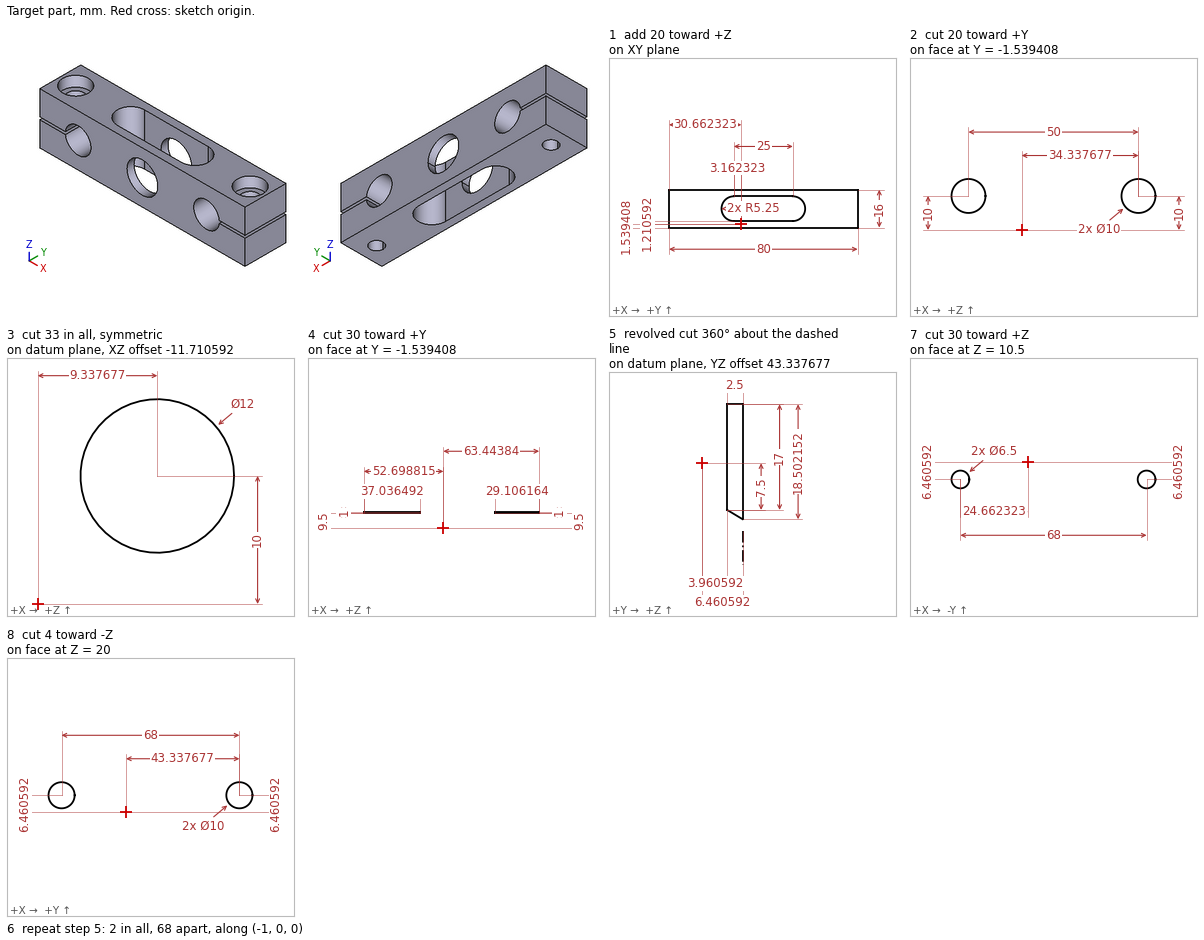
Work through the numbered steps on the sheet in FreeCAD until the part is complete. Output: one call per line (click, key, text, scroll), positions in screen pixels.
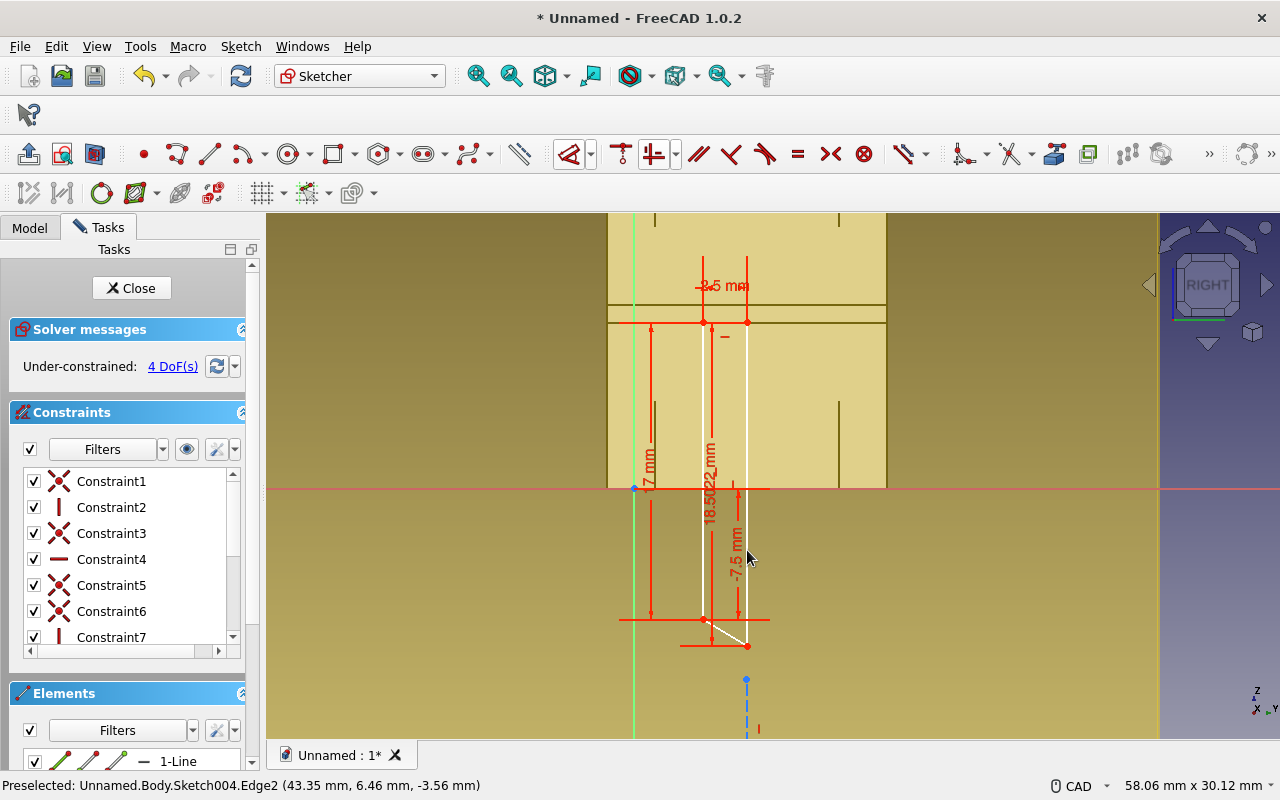
click(703, 620)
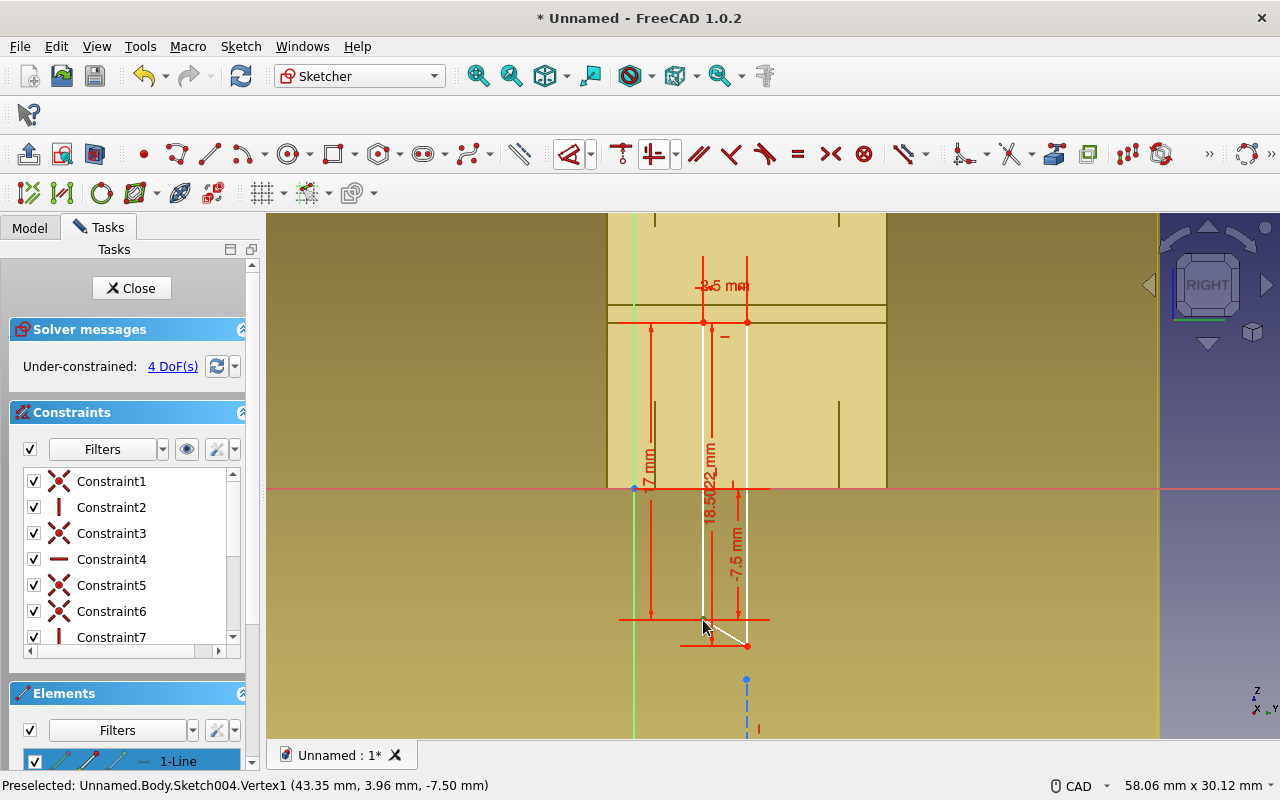
click(590, 154)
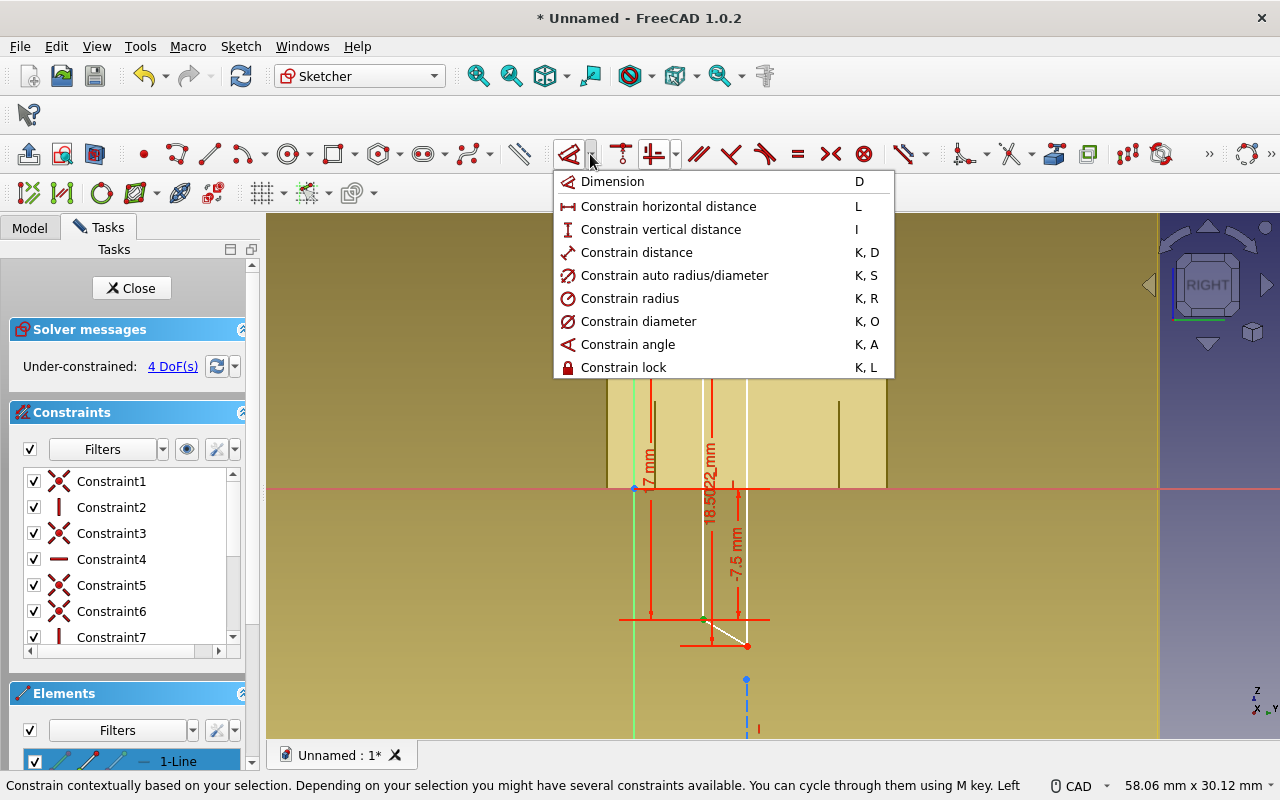
click(724, 206)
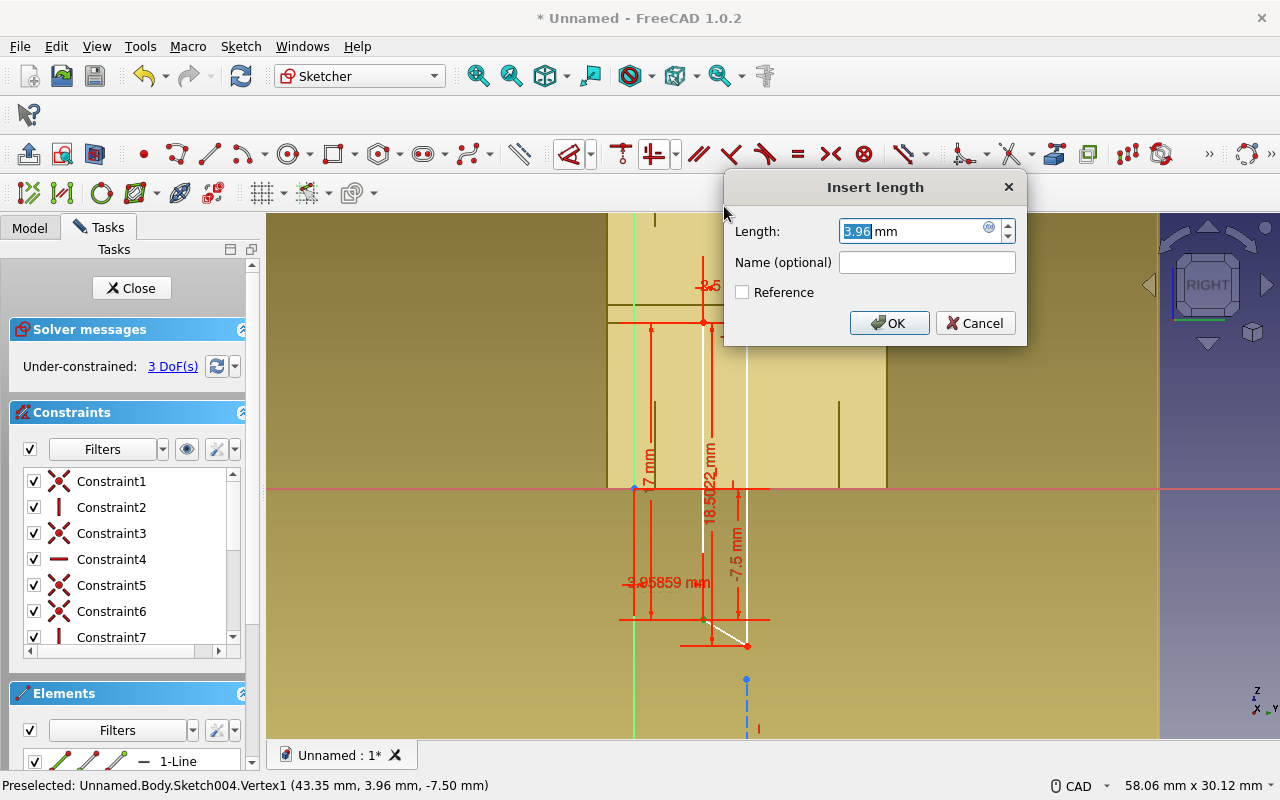
text(3.960592)
key(Return)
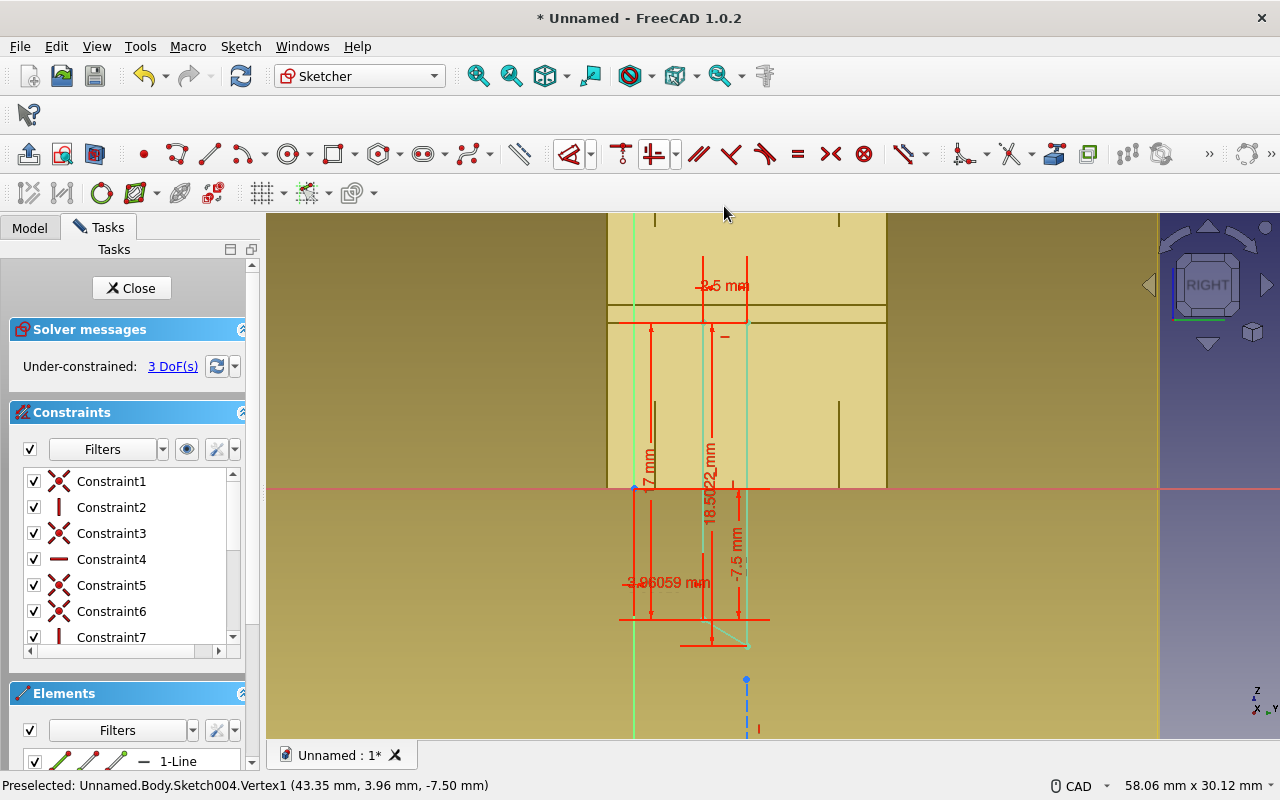
click(747, 680)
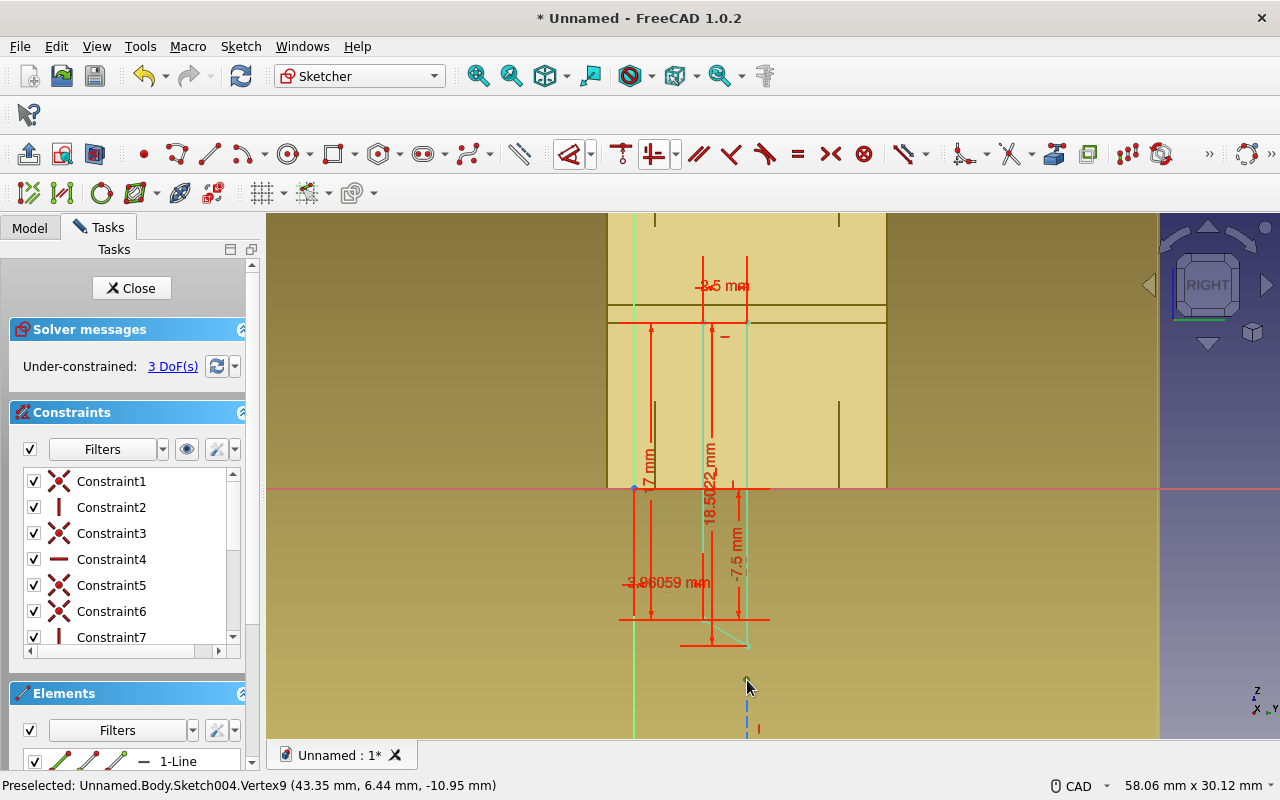
click(590, 154)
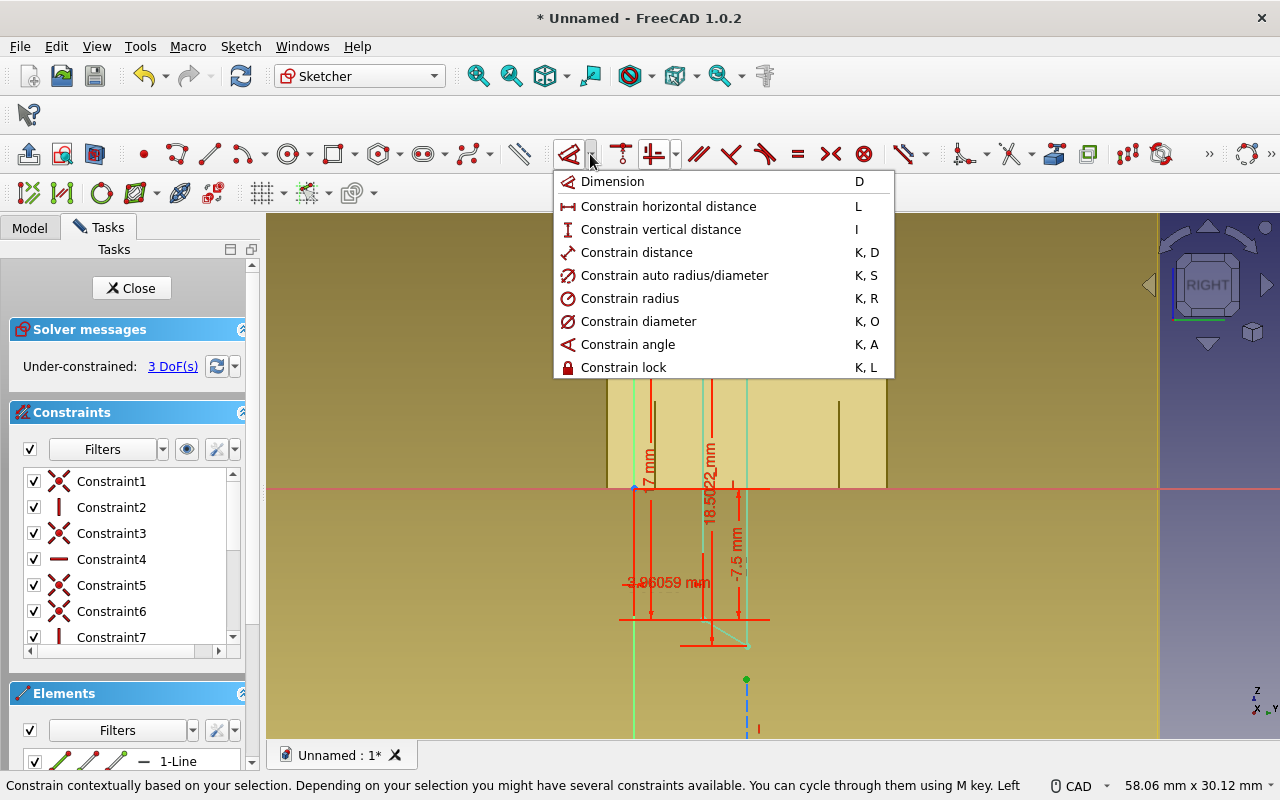
click(724, 206)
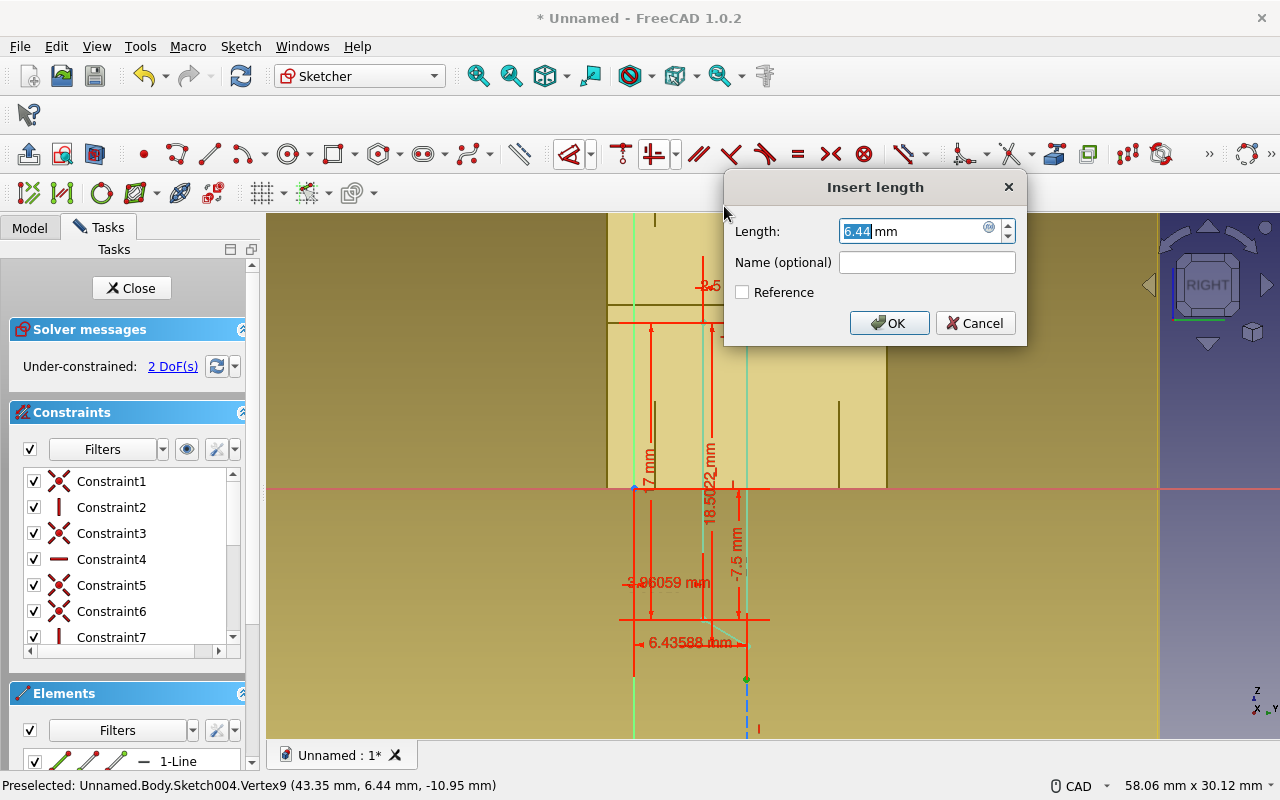
text(6.460592)
key(Return)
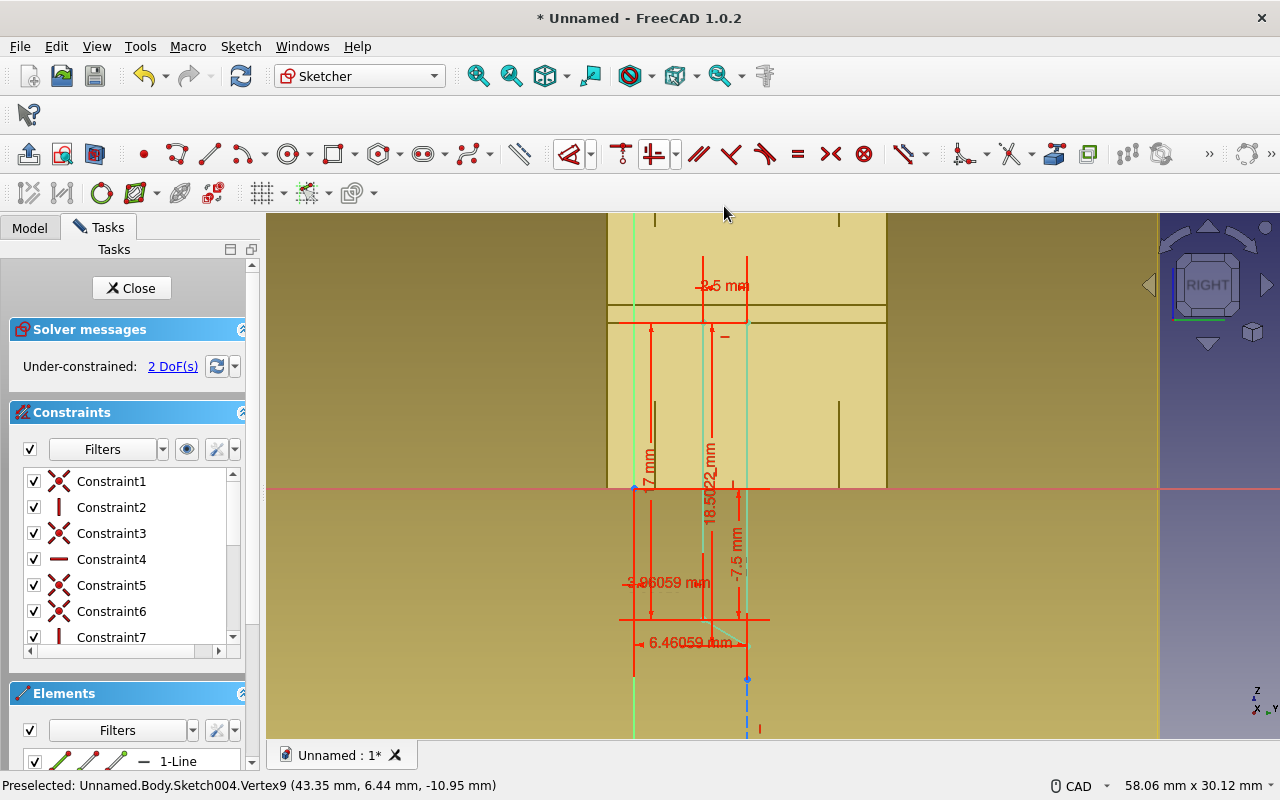
click(132, 288)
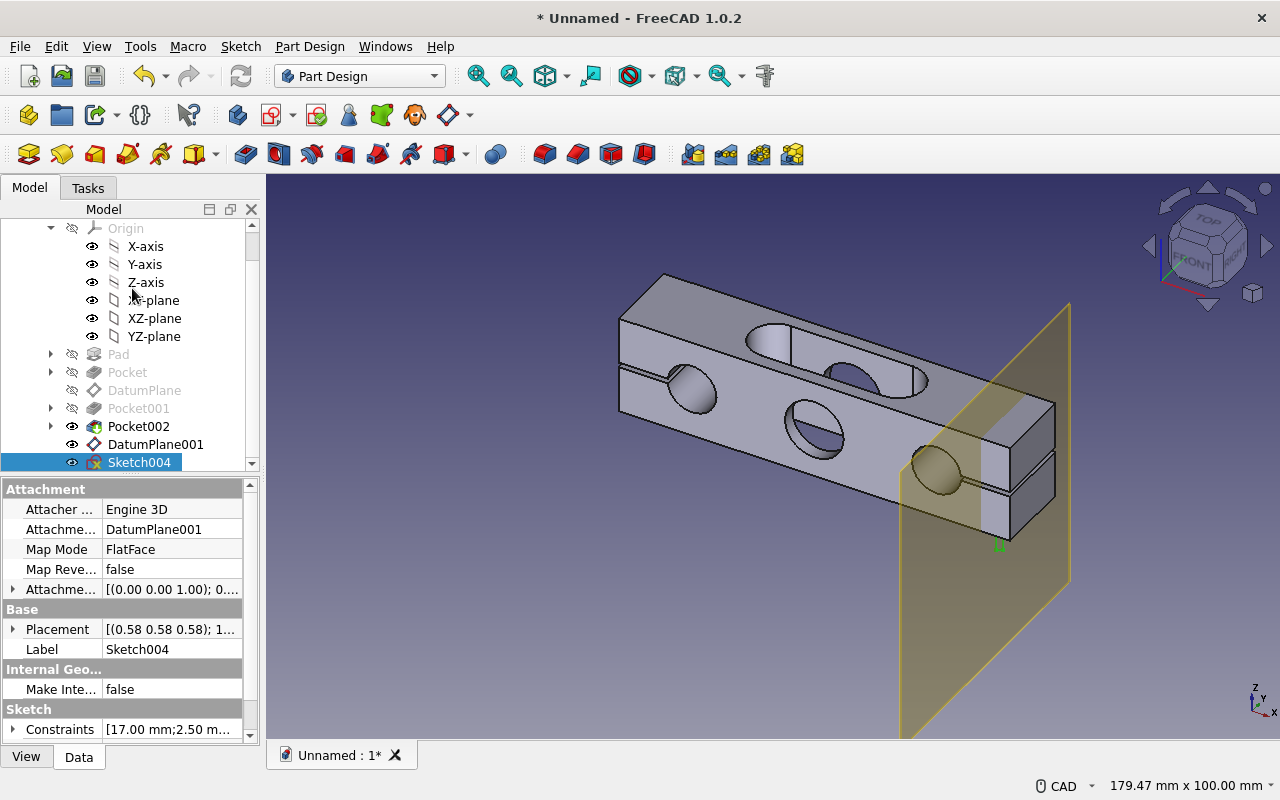
click(312, 154)